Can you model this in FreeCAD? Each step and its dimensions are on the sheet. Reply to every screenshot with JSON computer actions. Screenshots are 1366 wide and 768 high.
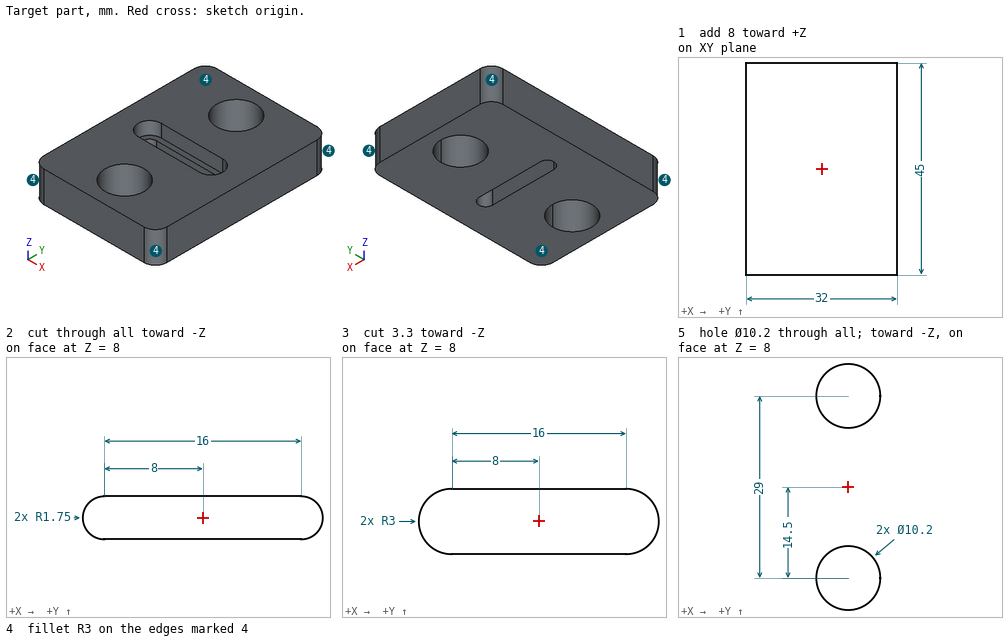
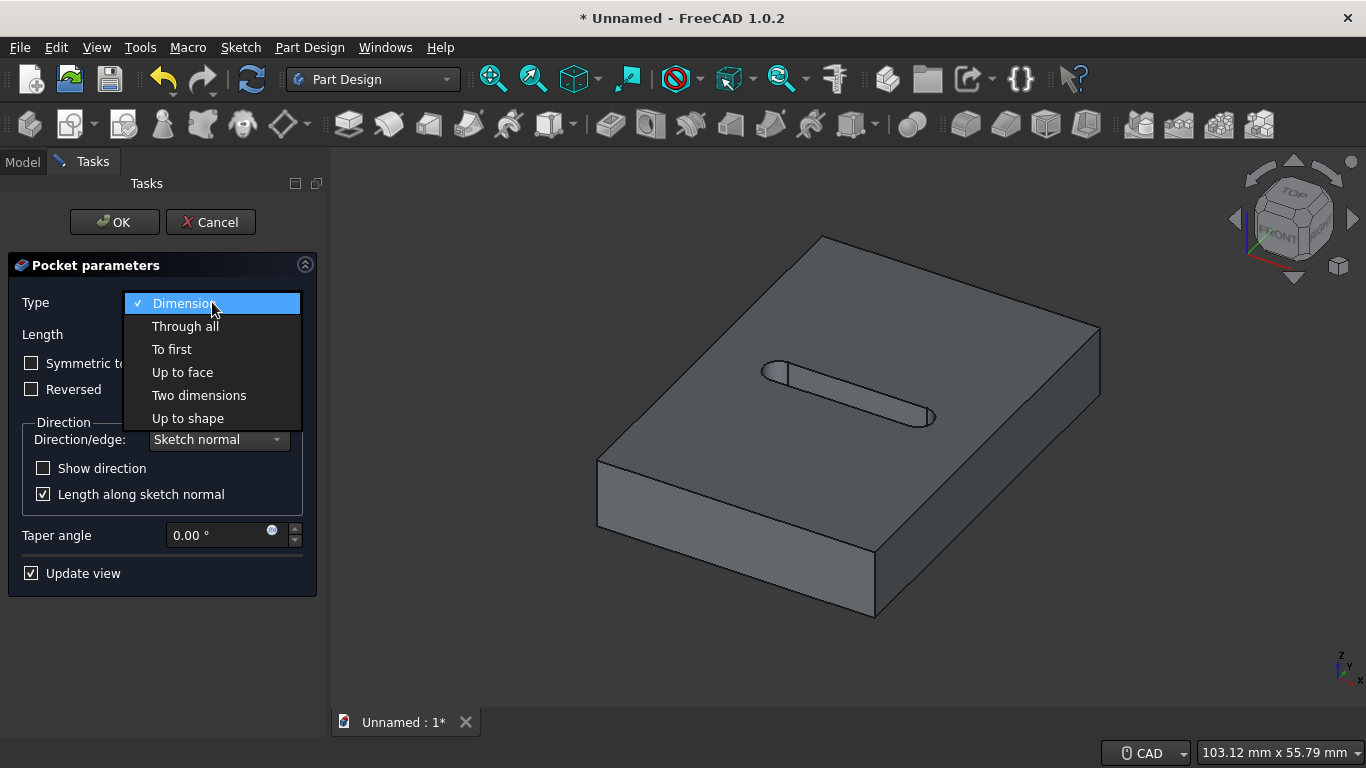
{"action": "left_click", "coordinate": [212, 326]}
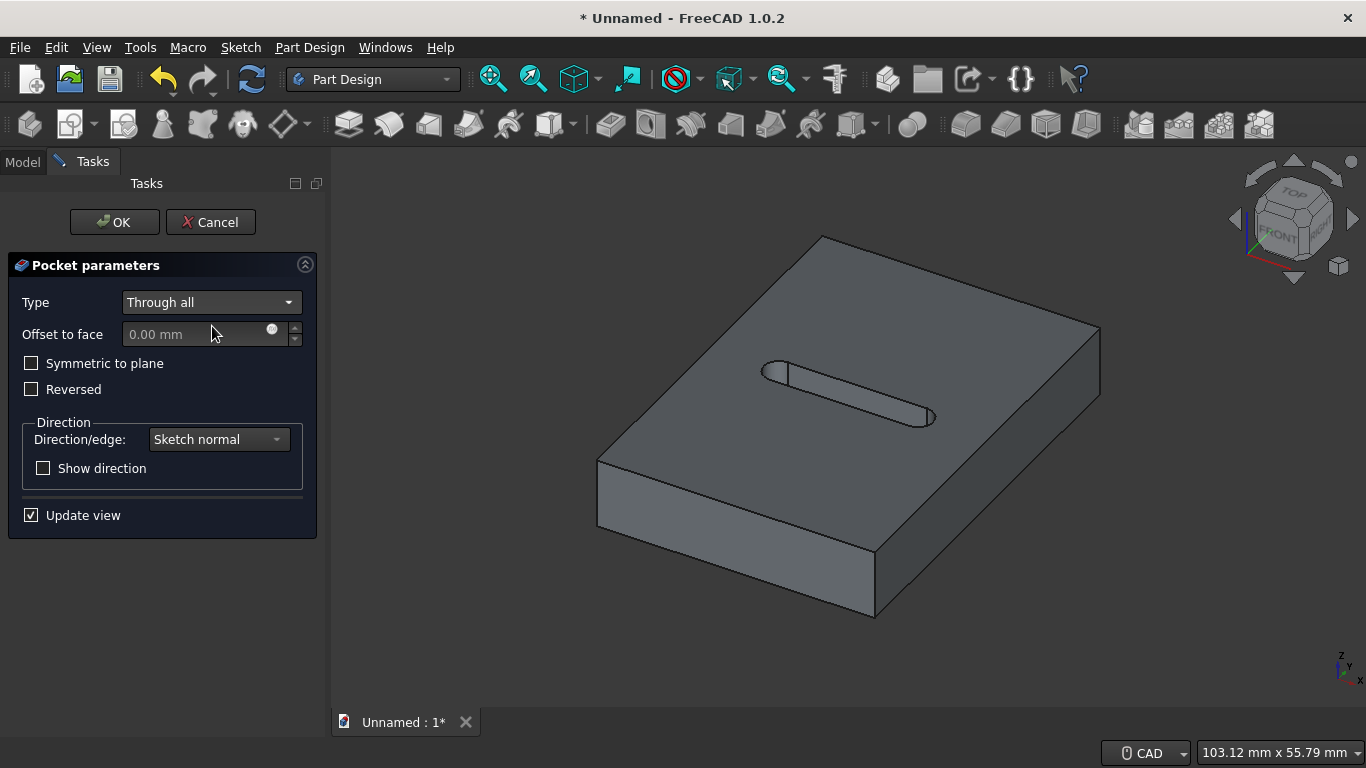
{"action": "left_click", "coordinate": [115, 222]}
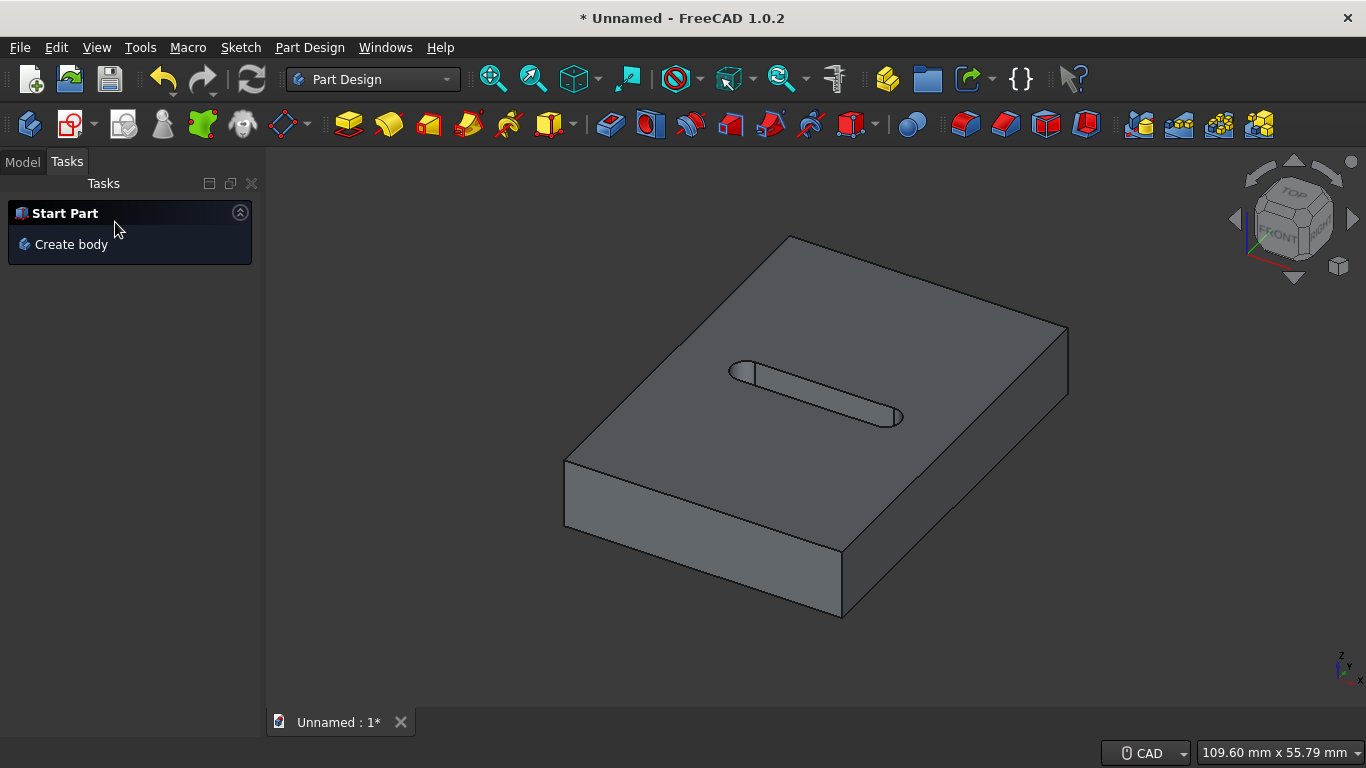
{"action": "left_click", "coordinate": [920, 342]}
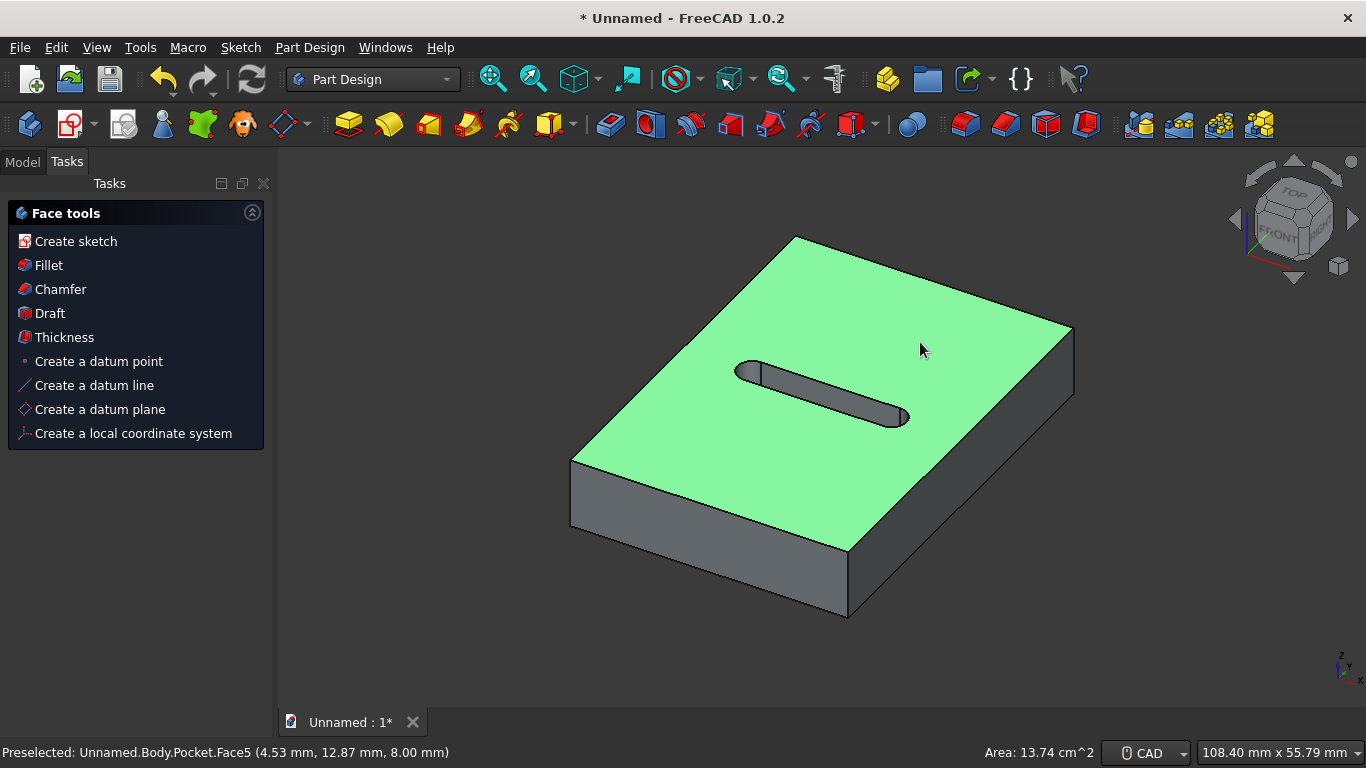
{"action": "left_click", "coordinate": [70, 124]}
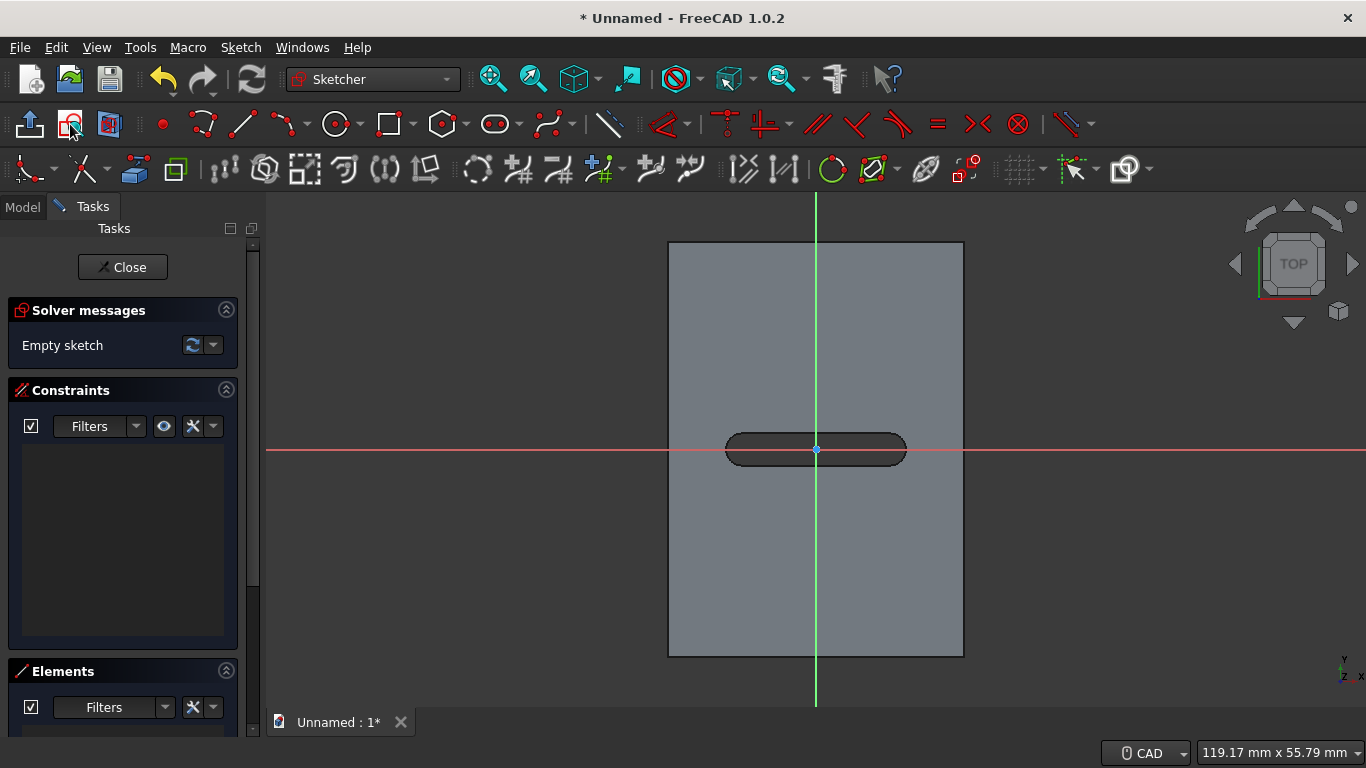
{"action": "scroll", "coordinate": [846, 449], "scroll_direction": "up", "scroll_amount": 6}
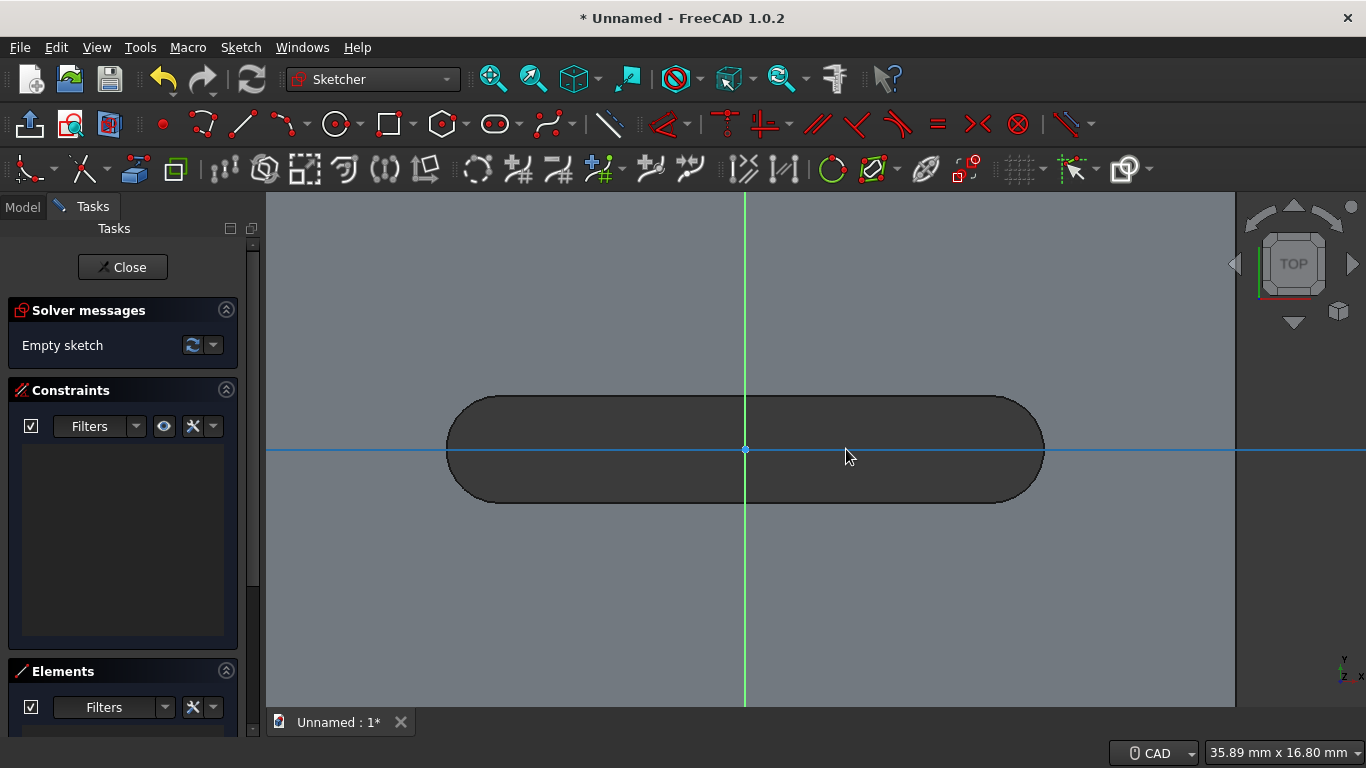
{"action": "key", "text": "g s"}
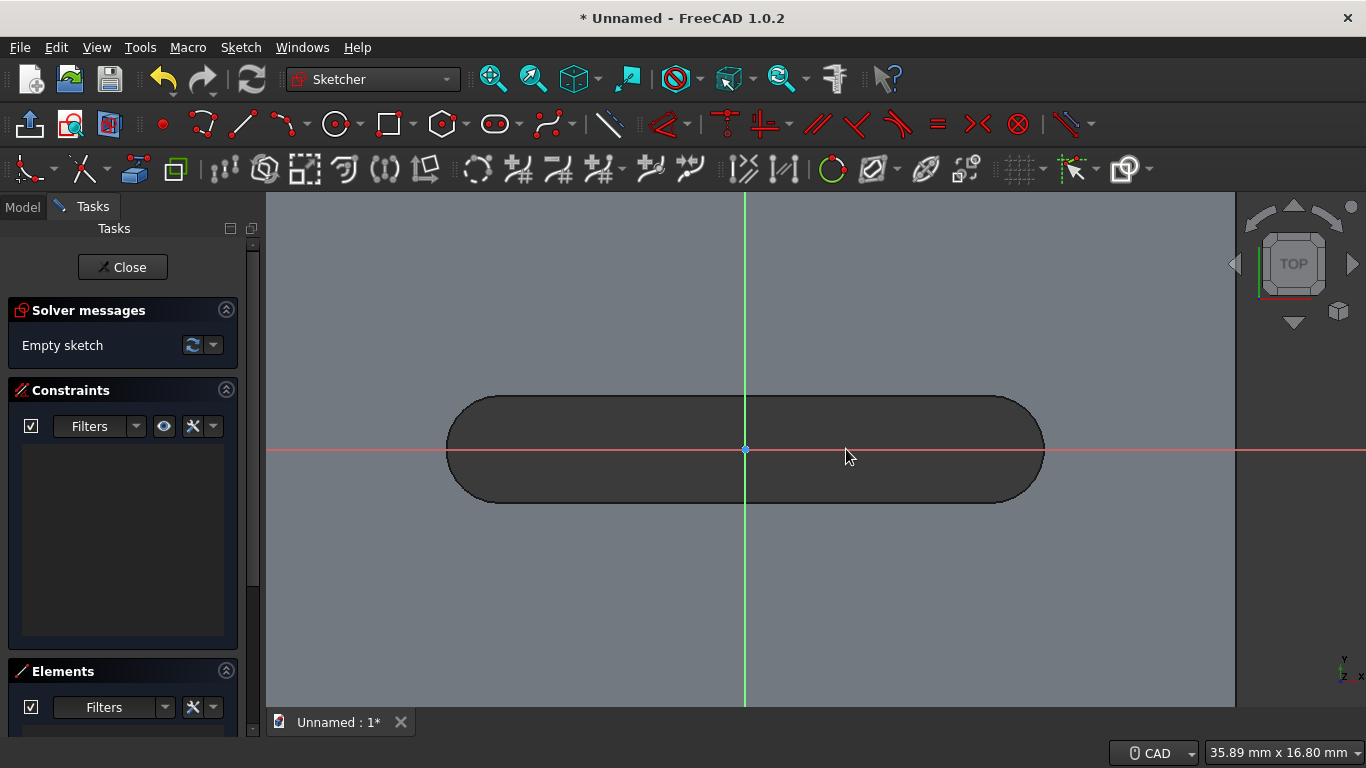
{"action": "left_click", "coordinate": [500, 450]}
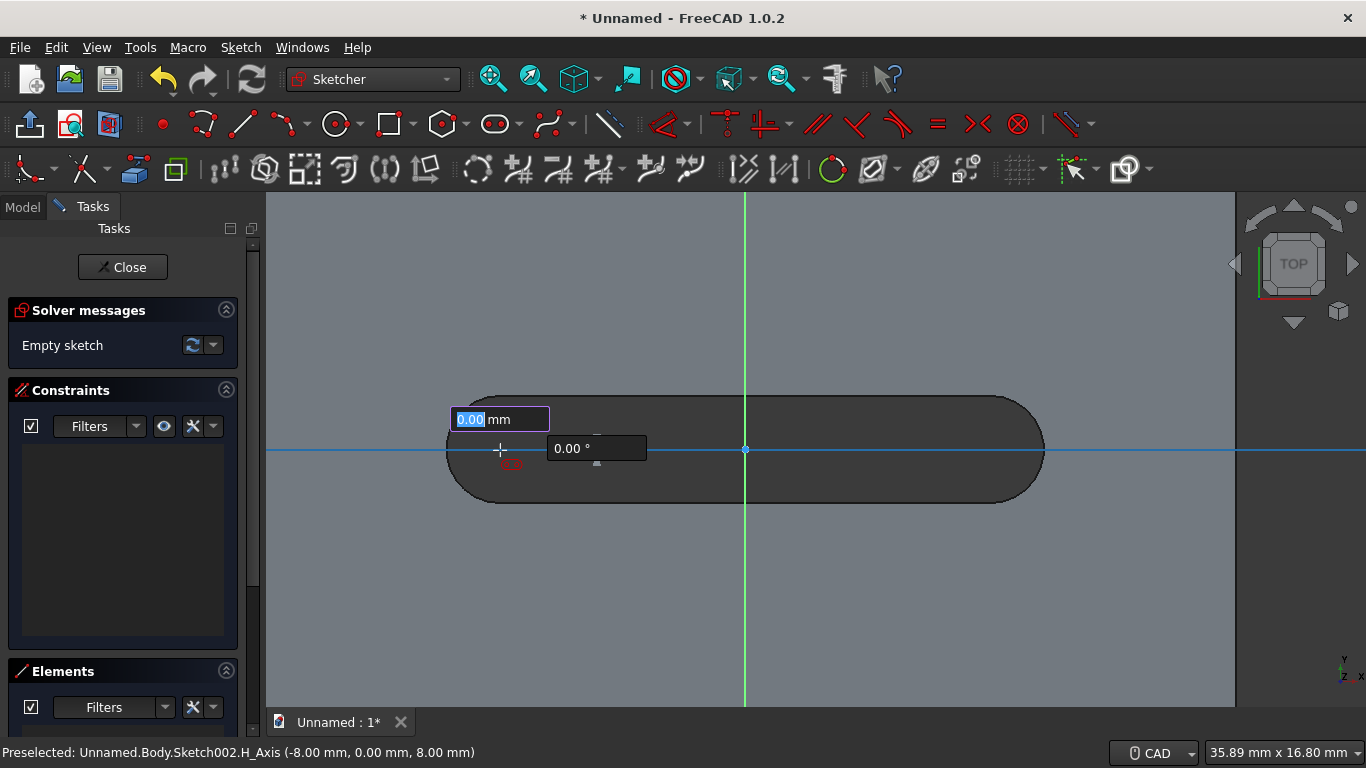
{"action": "left_click", "coordinate": [990, 440]}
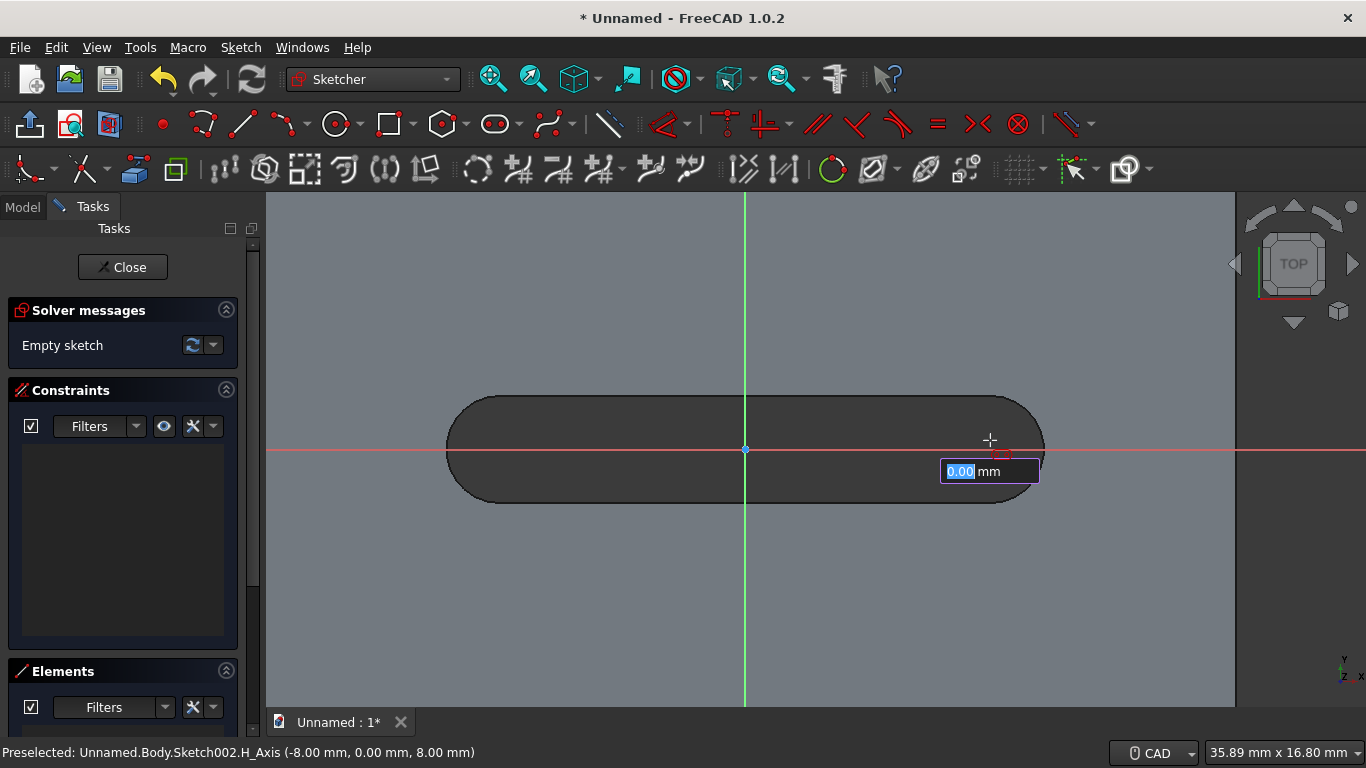
{"action": "left_click", "coordinate": [819, 358]}
{"action": "key", "text": "Escape"}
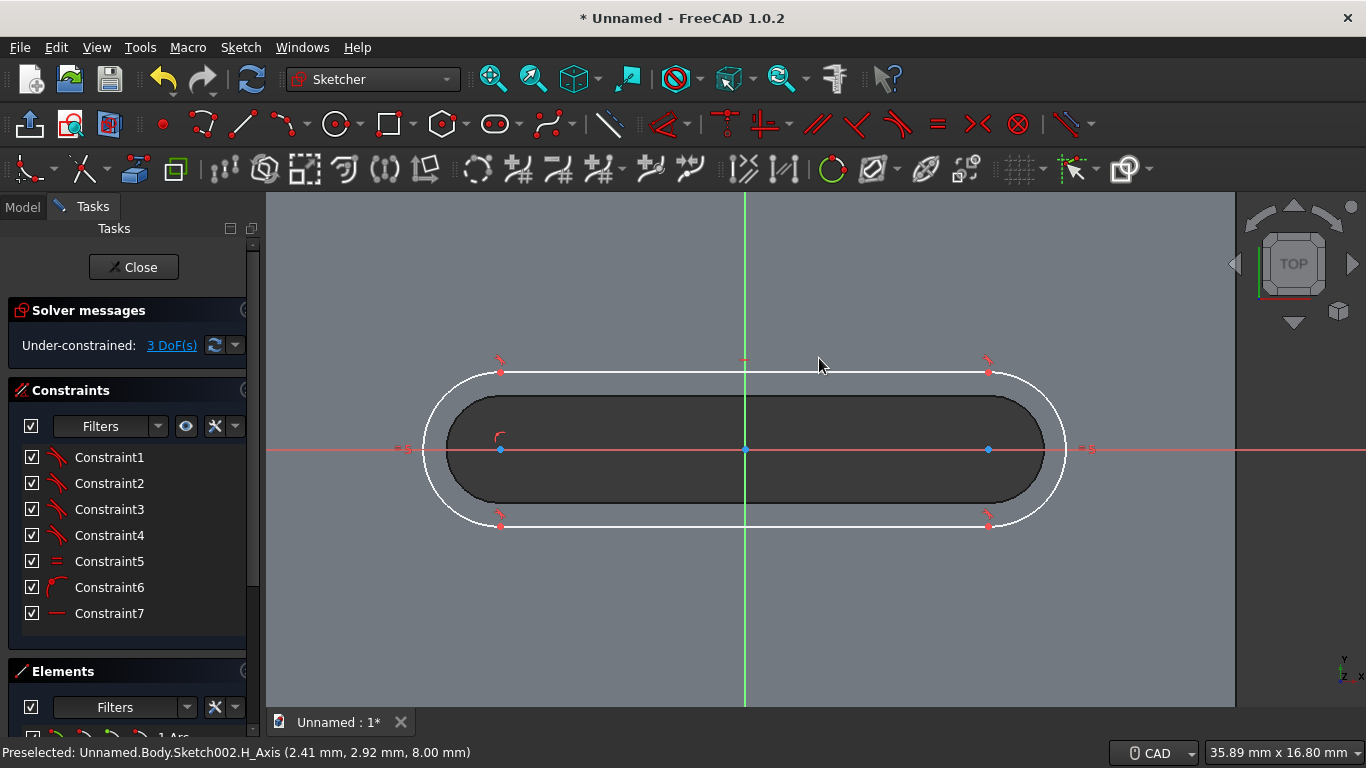
{"action": "key", "text": "d"}